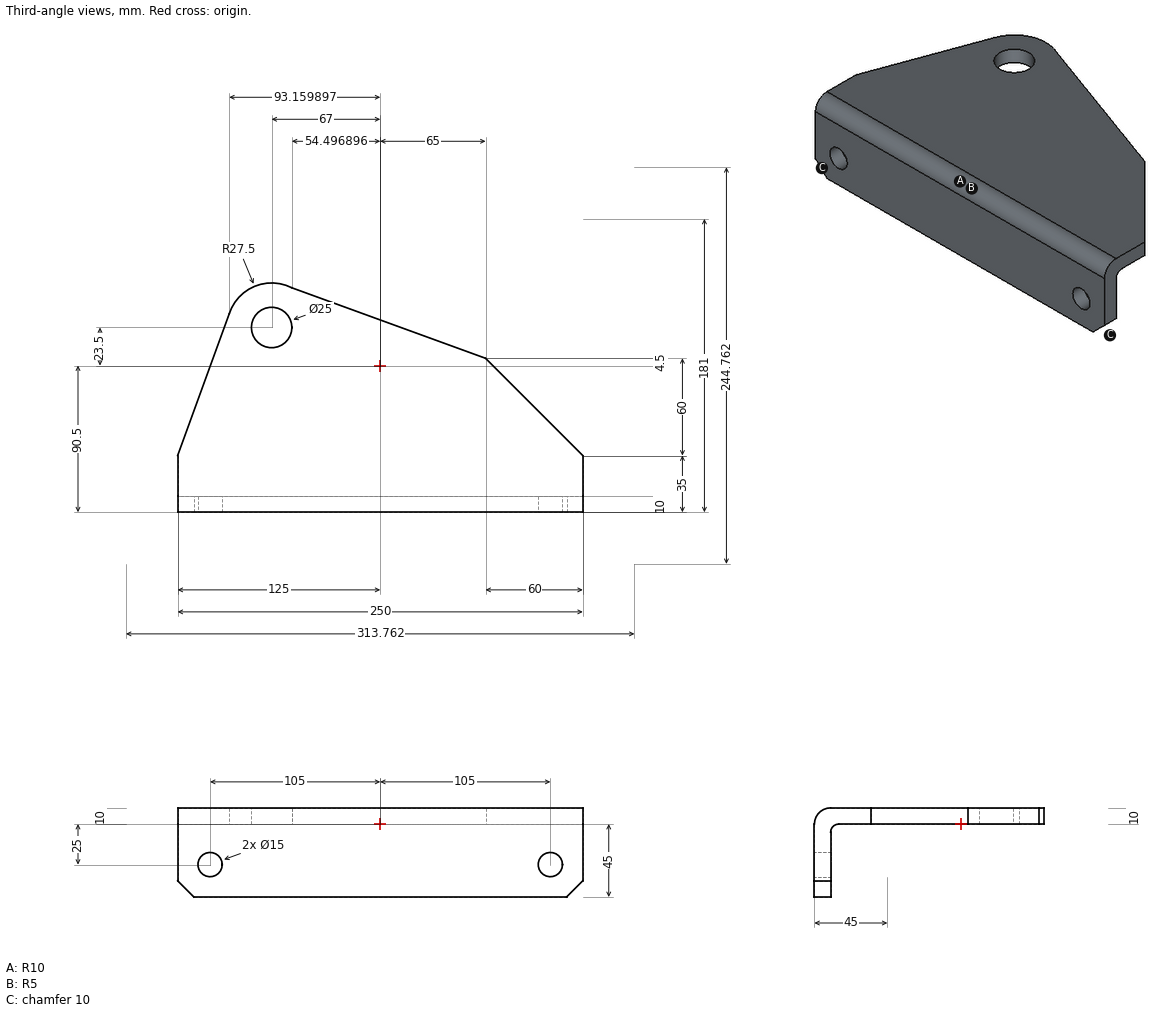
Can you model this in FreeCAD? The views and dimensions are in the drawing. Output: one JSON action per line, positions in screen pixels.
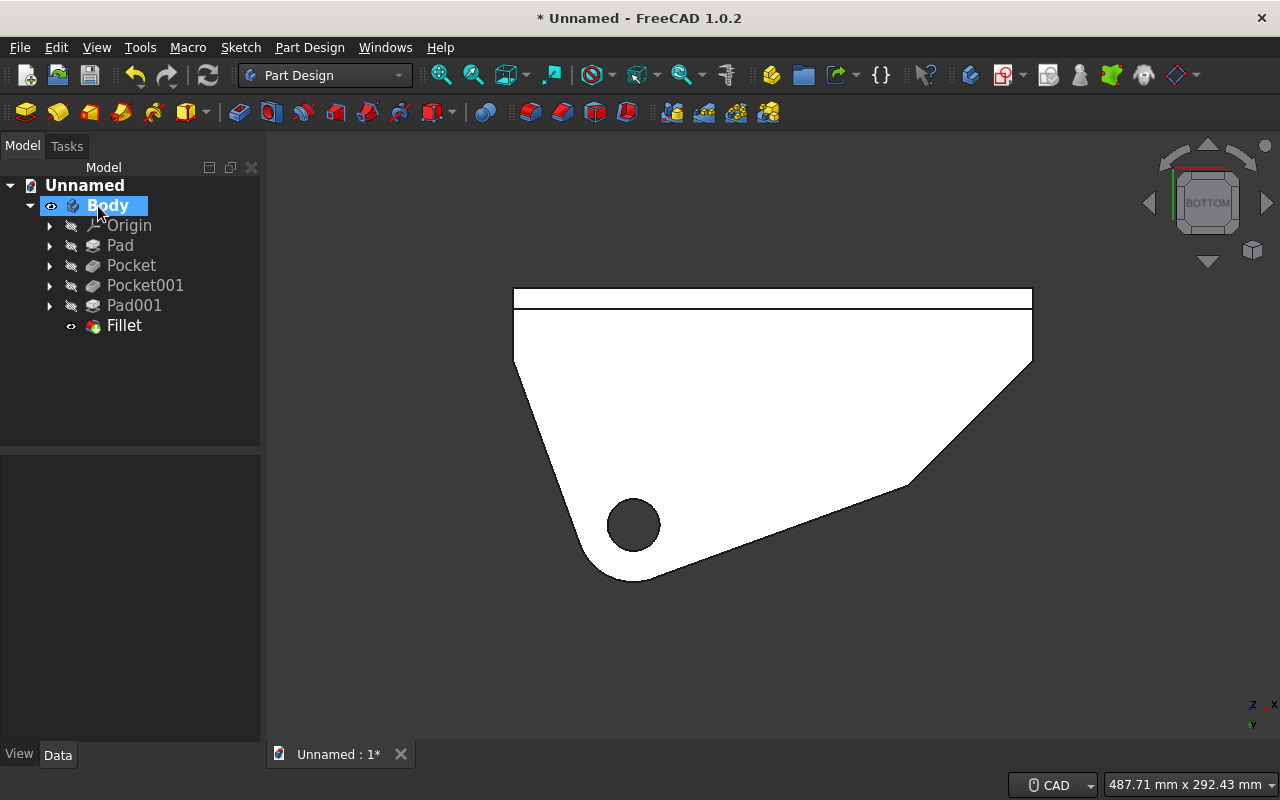
{"action": "key", "text": "4"}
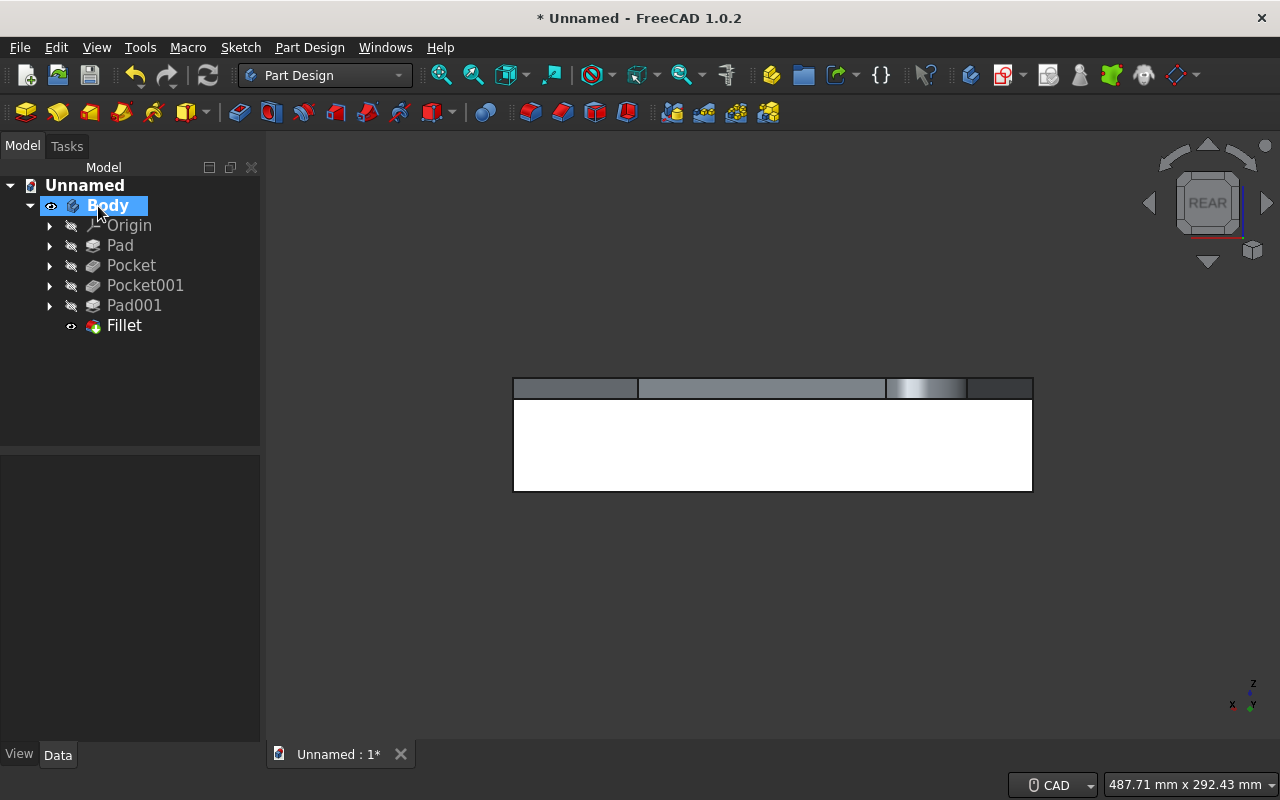
{"action": "key", "text": "6"}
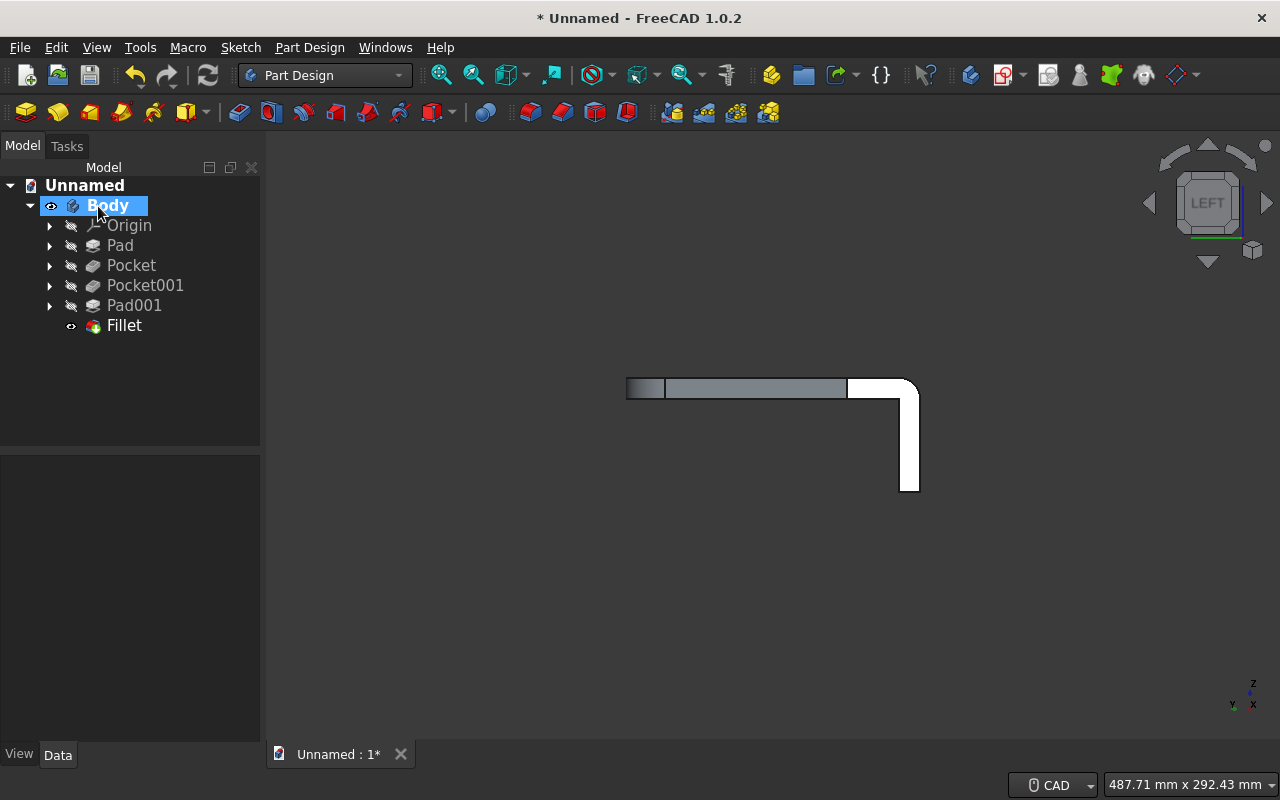
{"action": "left_click", "coordinate": [442, 76]}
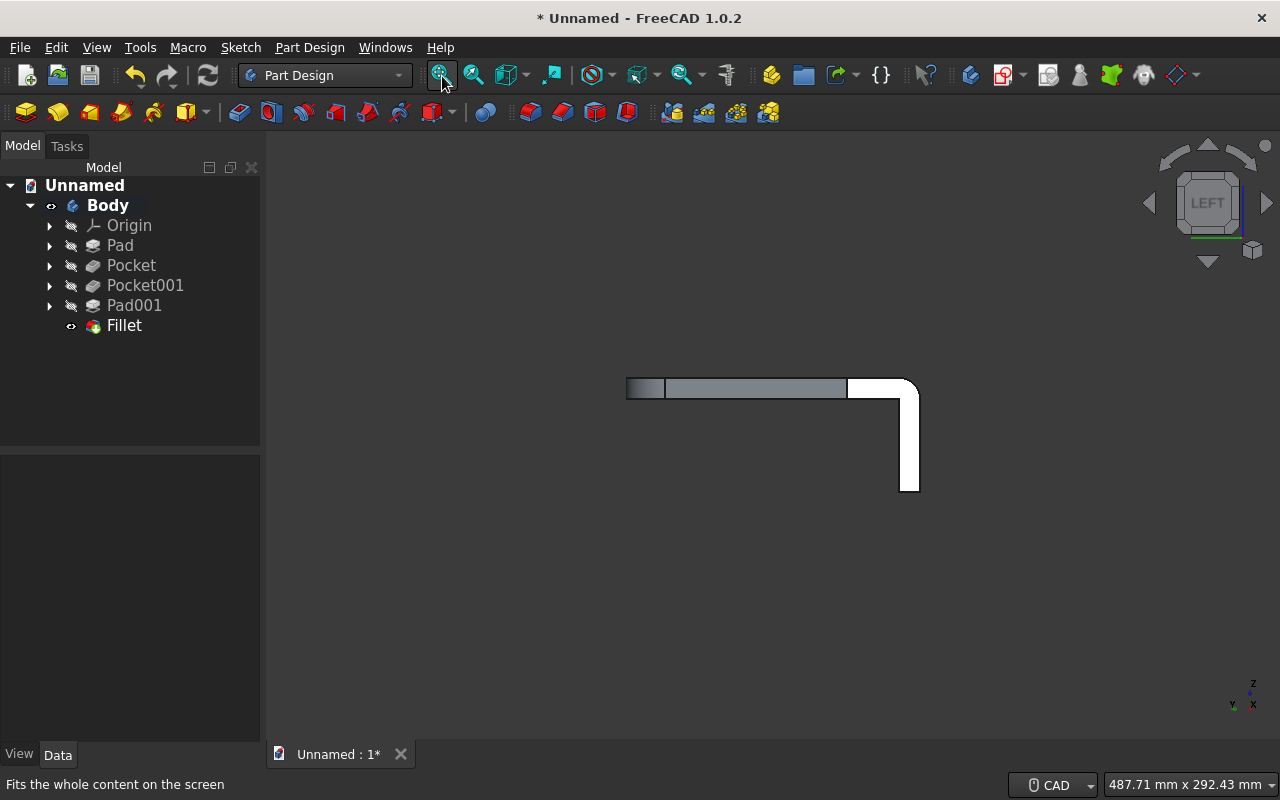
{"action": "key", "text": "v 3"}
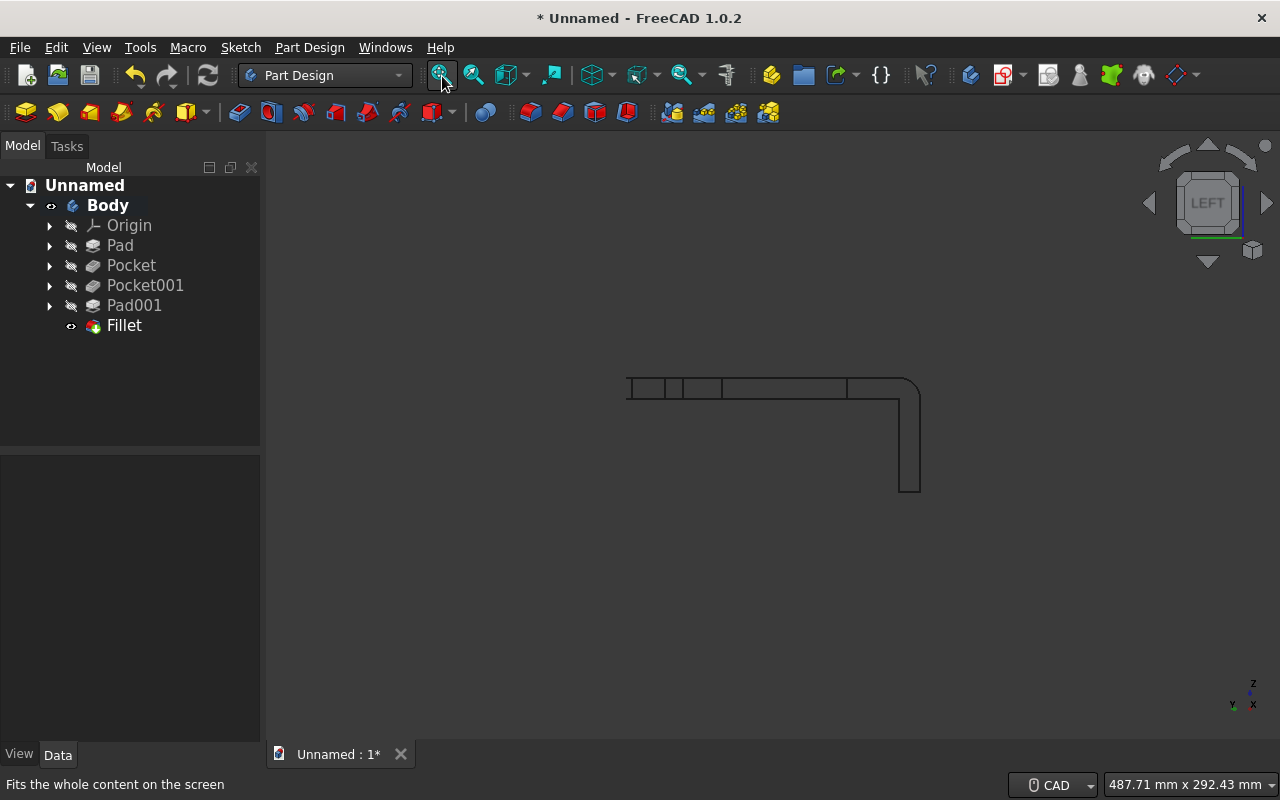
{"action": "key", "text": "0"}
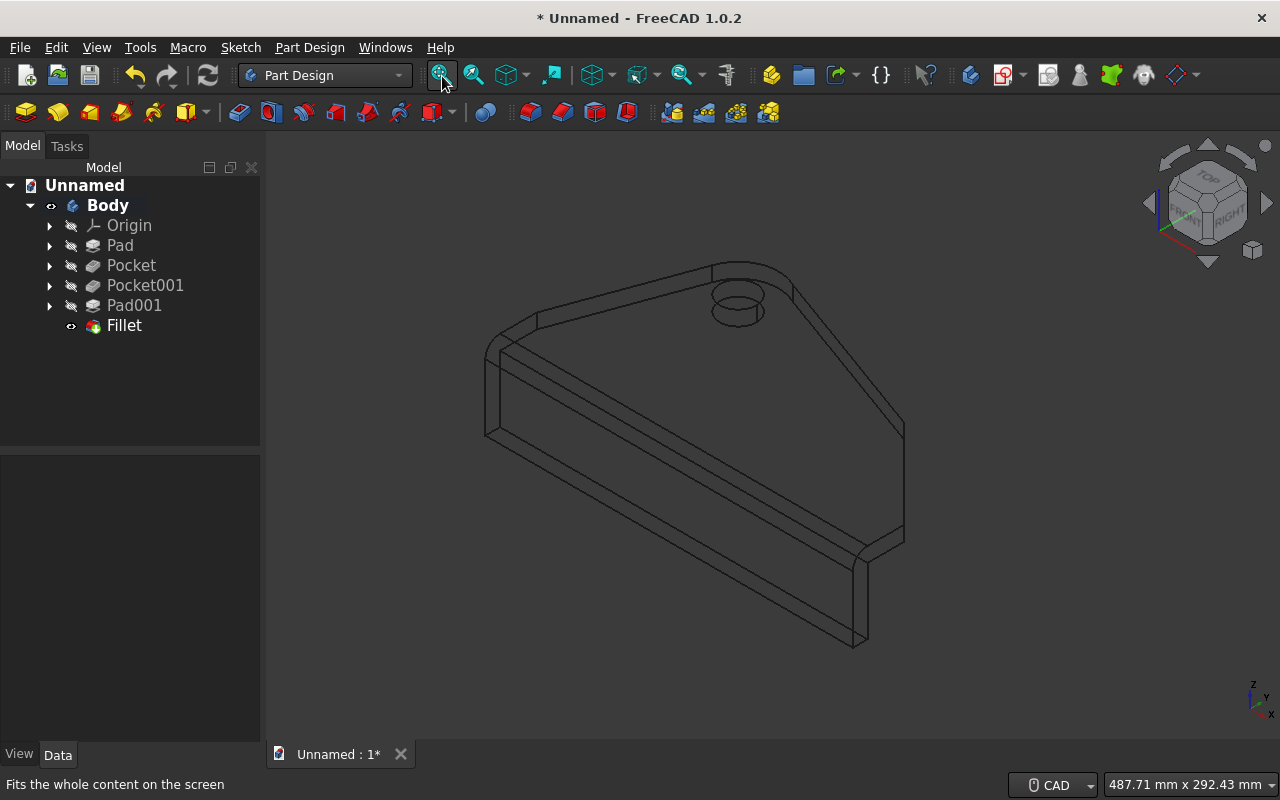
{"action": "left_click", "coordinate": [684, 456]}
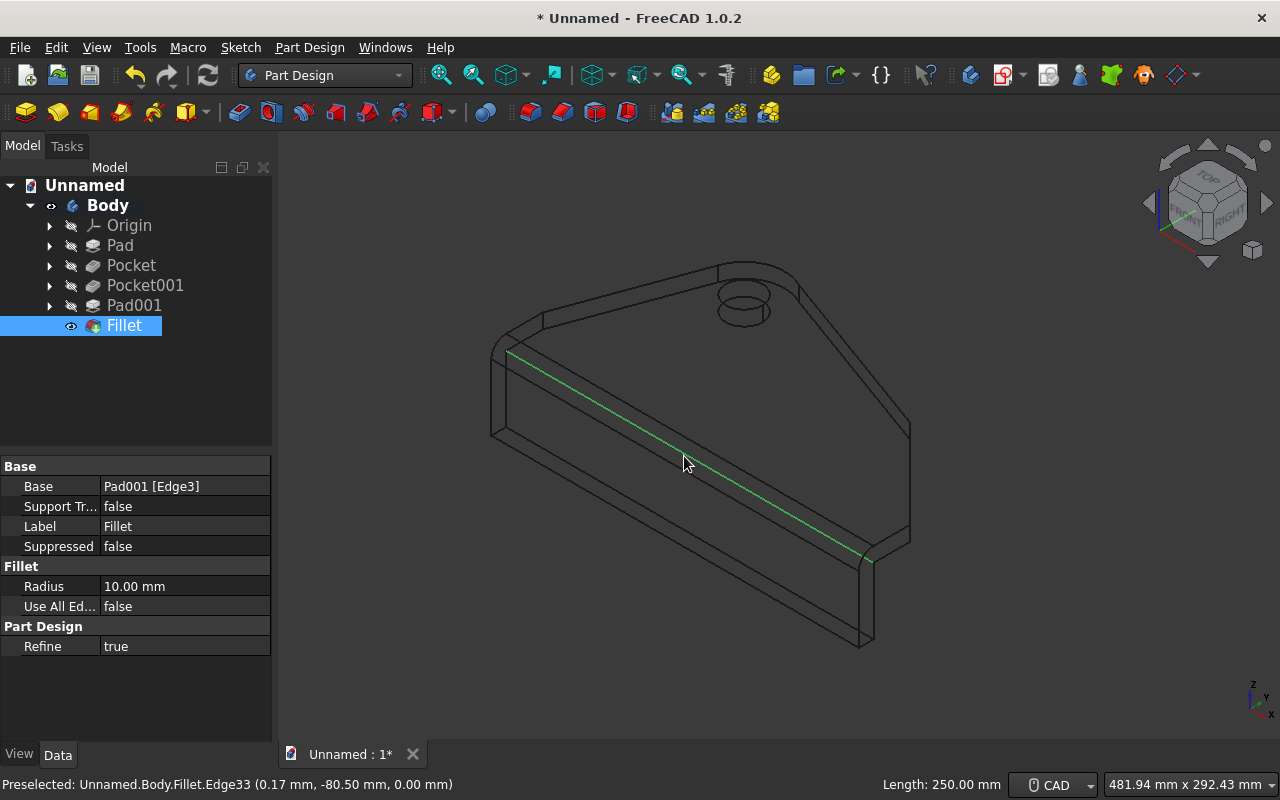
{"action": "key", "text": "v 1"}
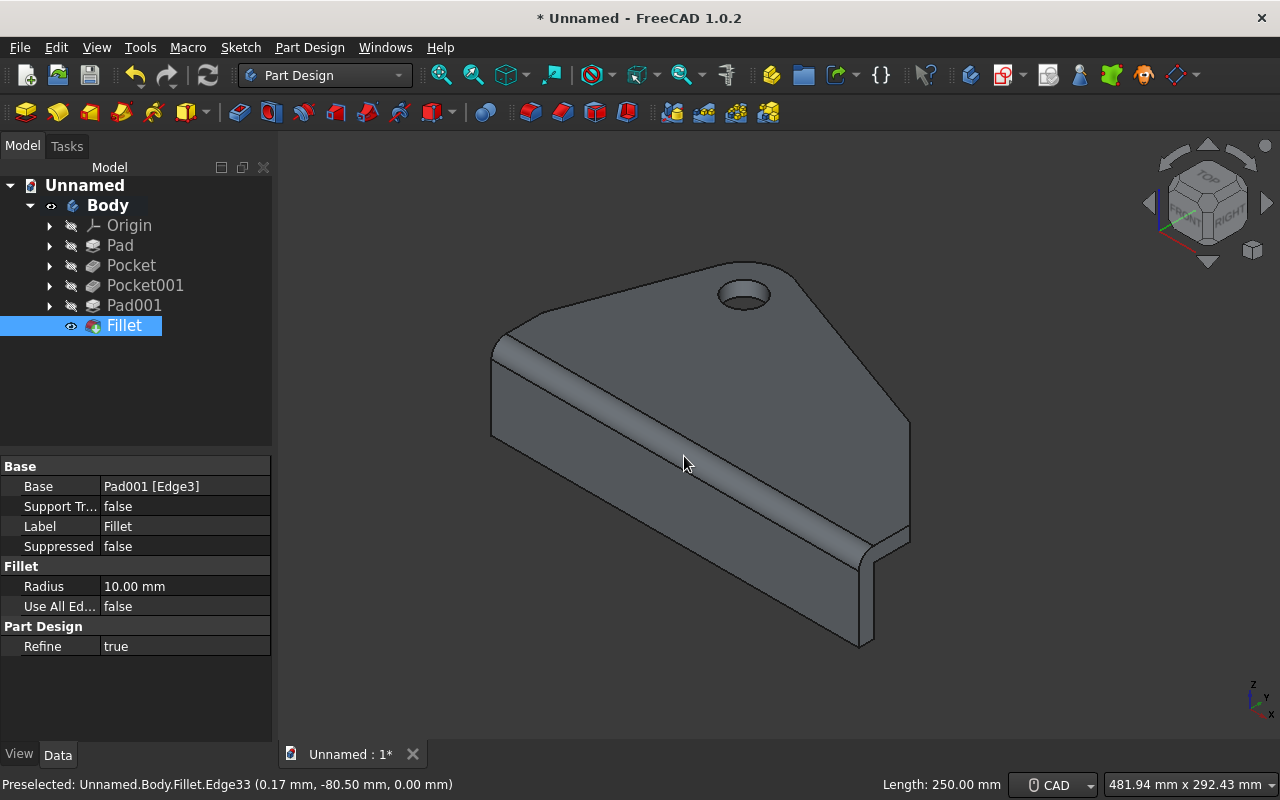
{"action": "left_click", "coordinate": [532, 112]}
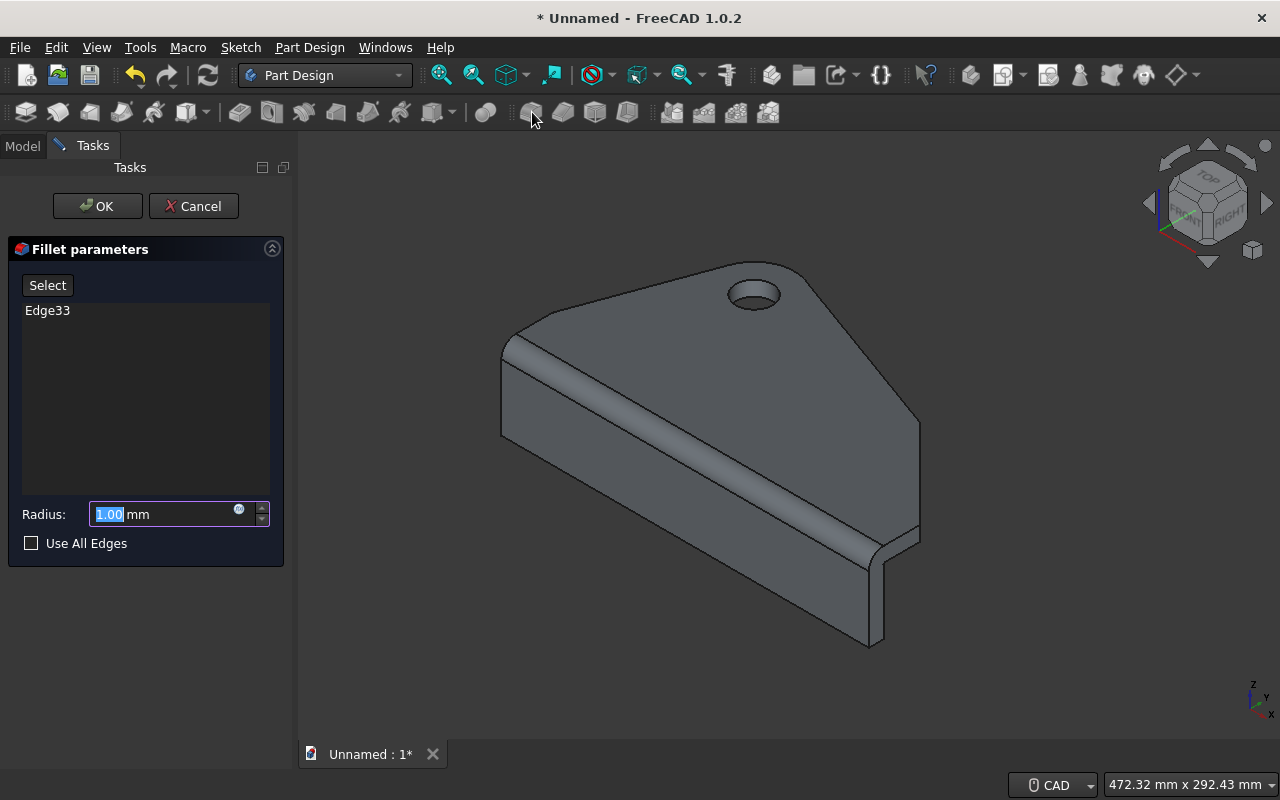
{"action": "type", "text": "5"}
{"action": "key", "text": "Tab"}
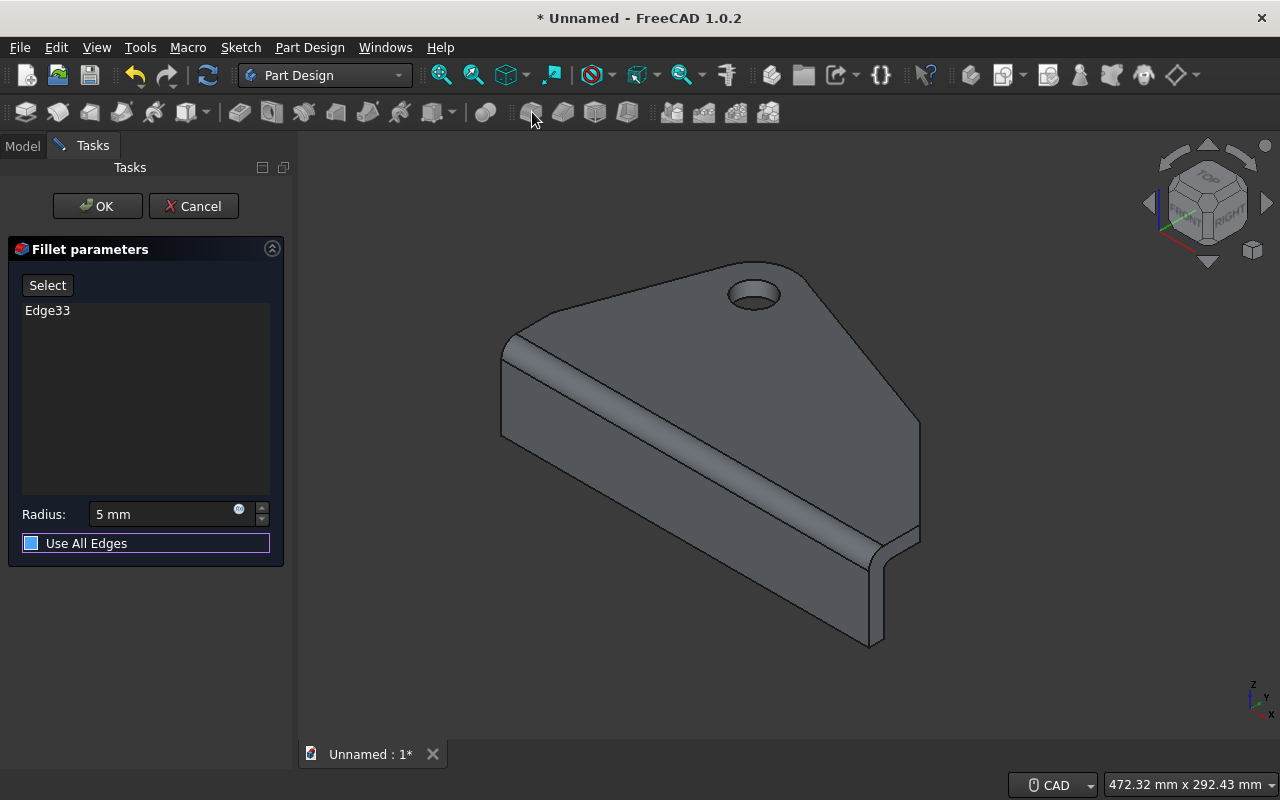
{"action": "left_click", "coordinate": [98, 206]}